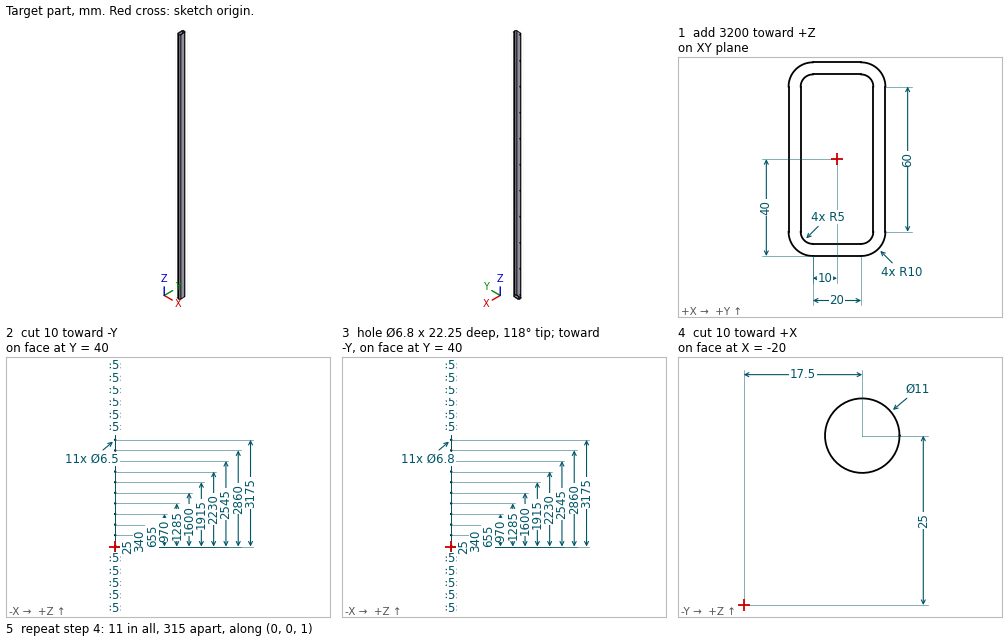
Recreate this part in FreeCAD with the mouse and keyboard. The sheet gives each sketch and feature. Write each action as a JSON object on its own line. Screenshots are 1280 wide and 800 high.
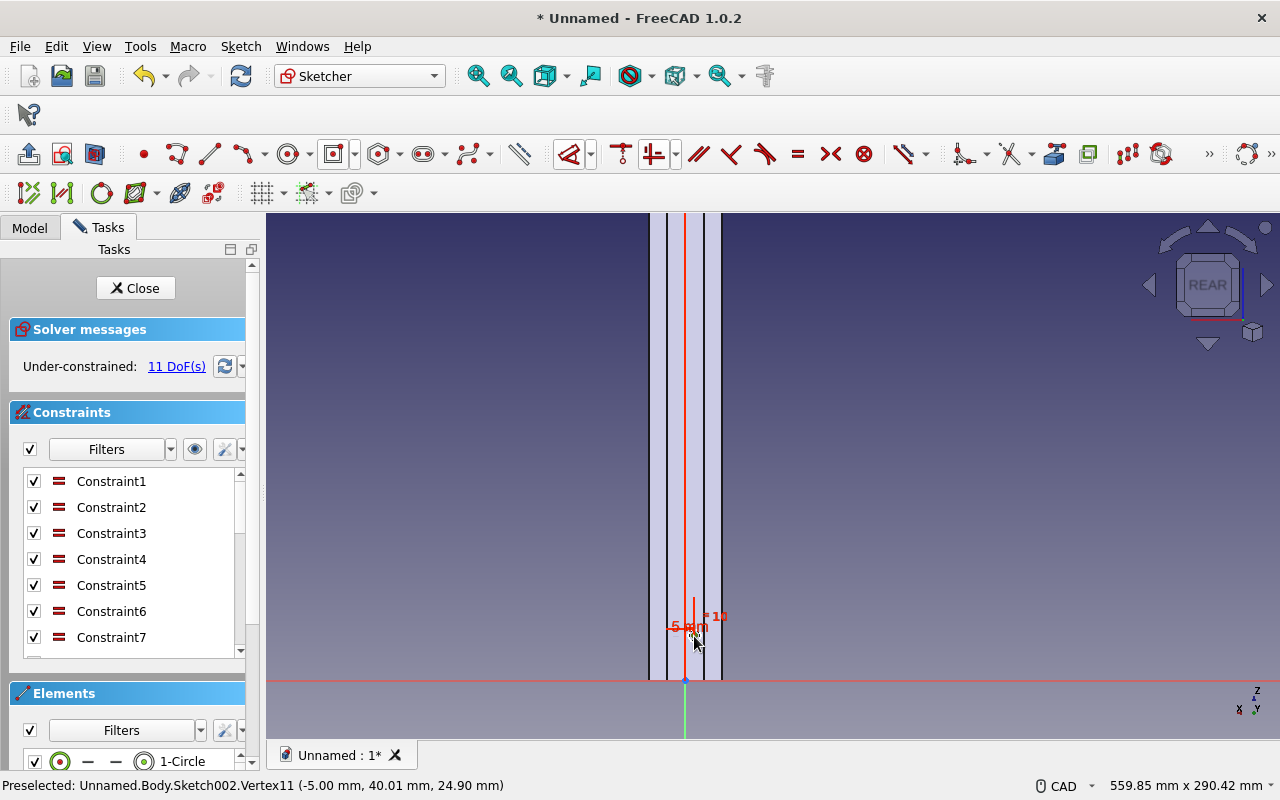
{"action": "key", "text": "i"}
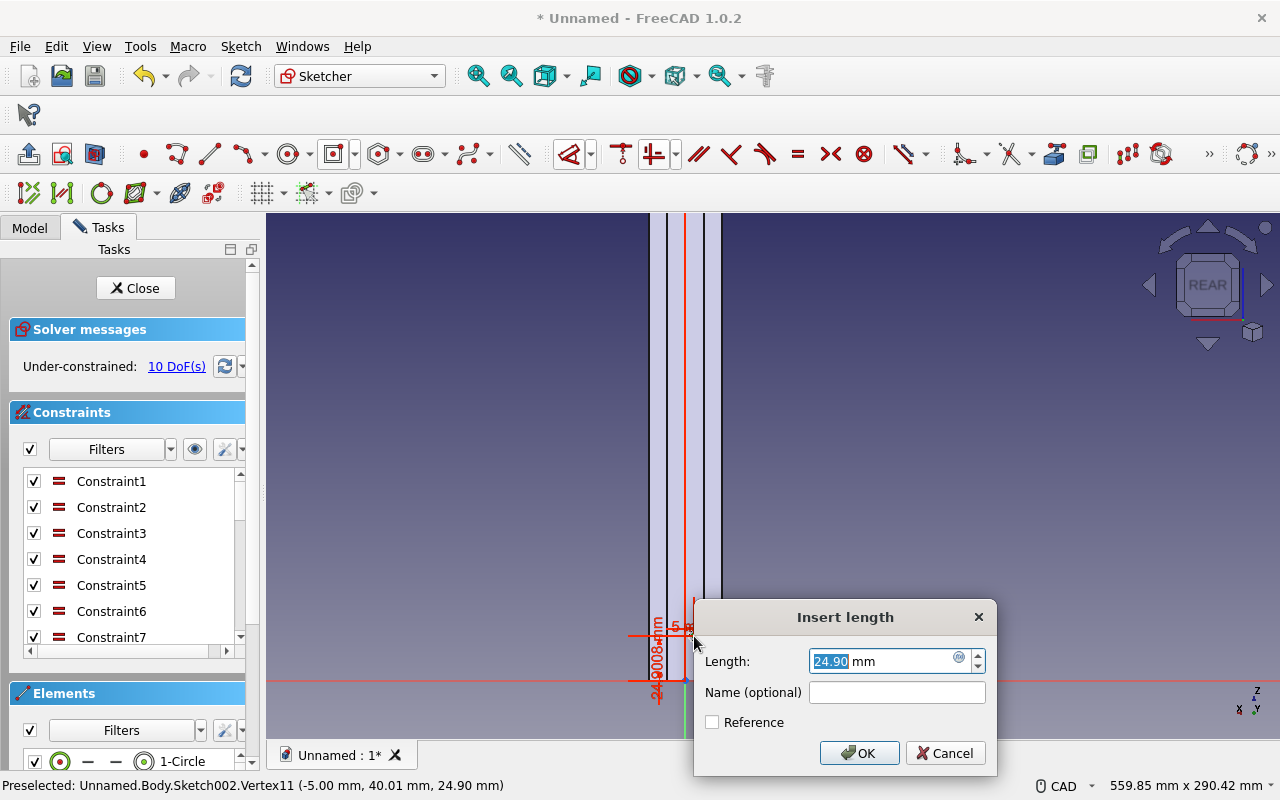
{"action": "type", "text": "25"}
{"action": "key", "text": "Return"}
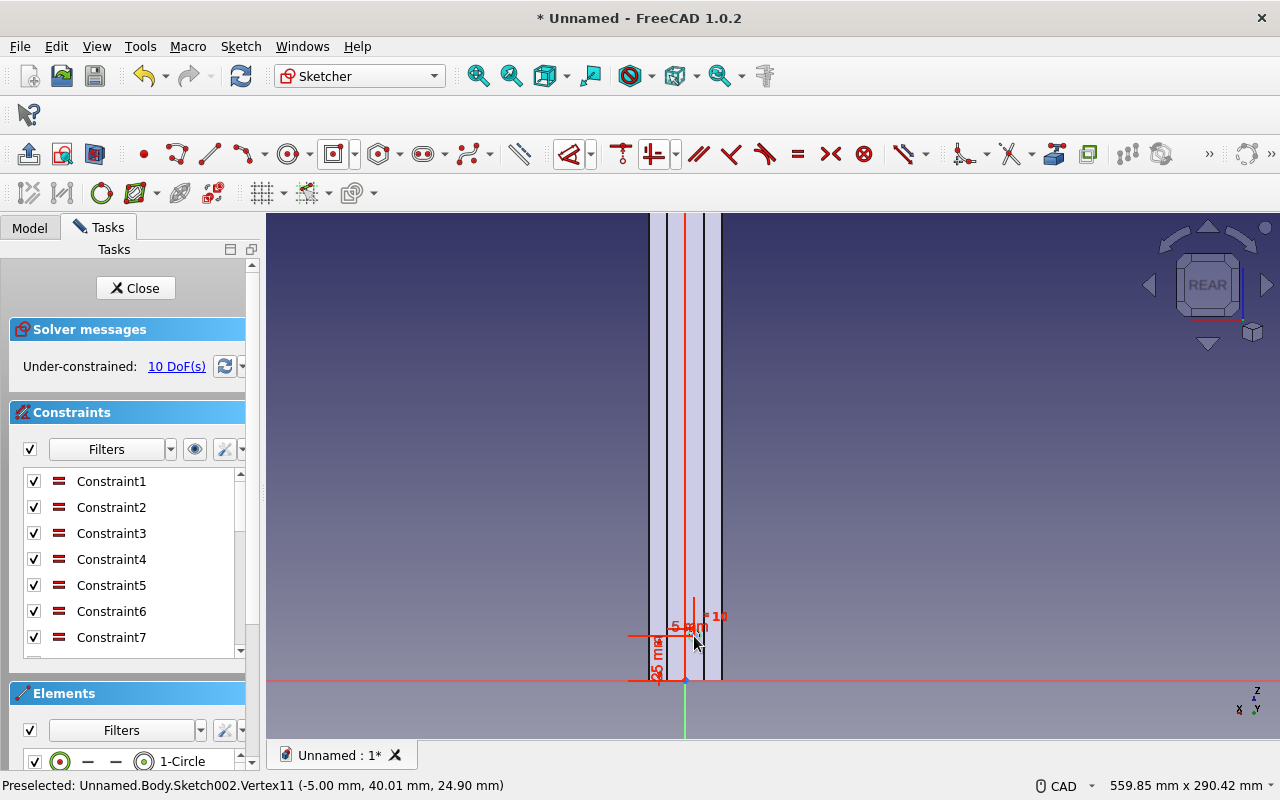
{"action": "scroll", "coordinate": [705, 649], "scroll_direction": "down", "scroll_amount": 14}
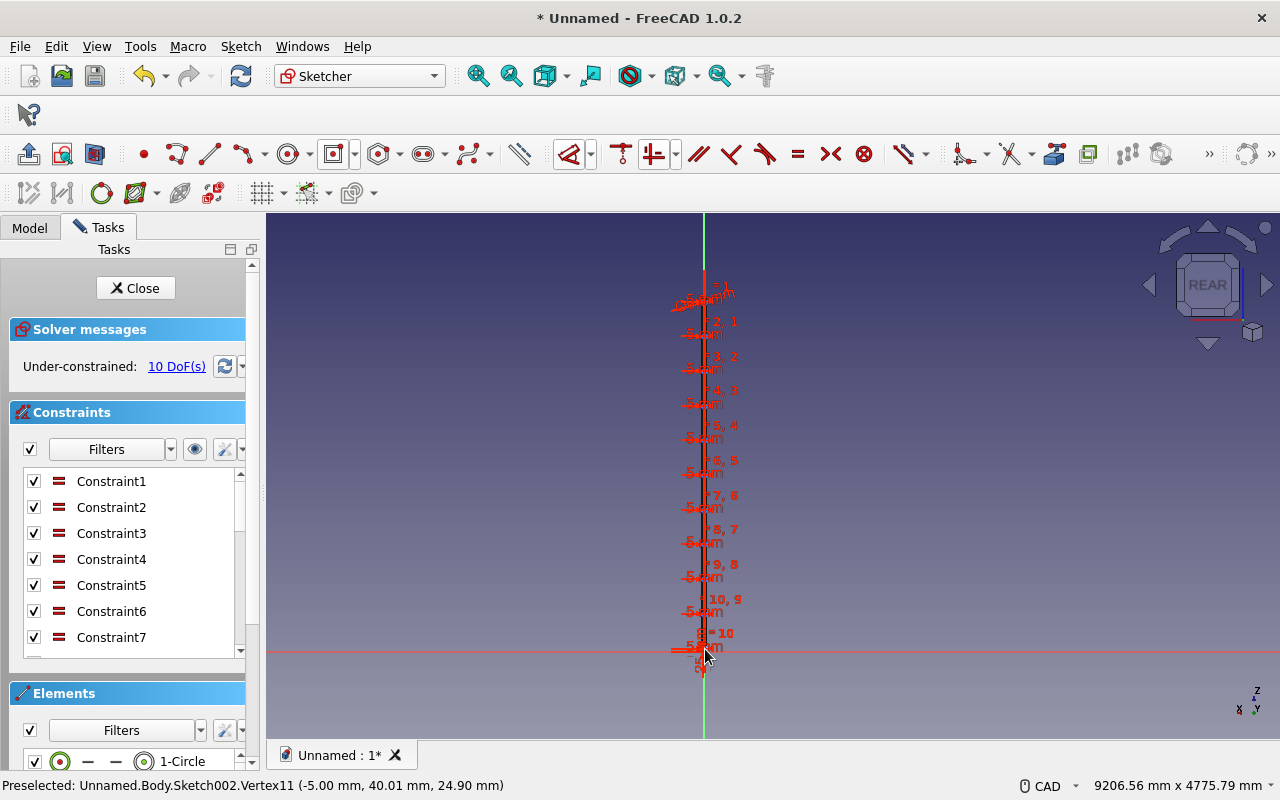
{"action": "left_click", "coordinate": [705, 545]}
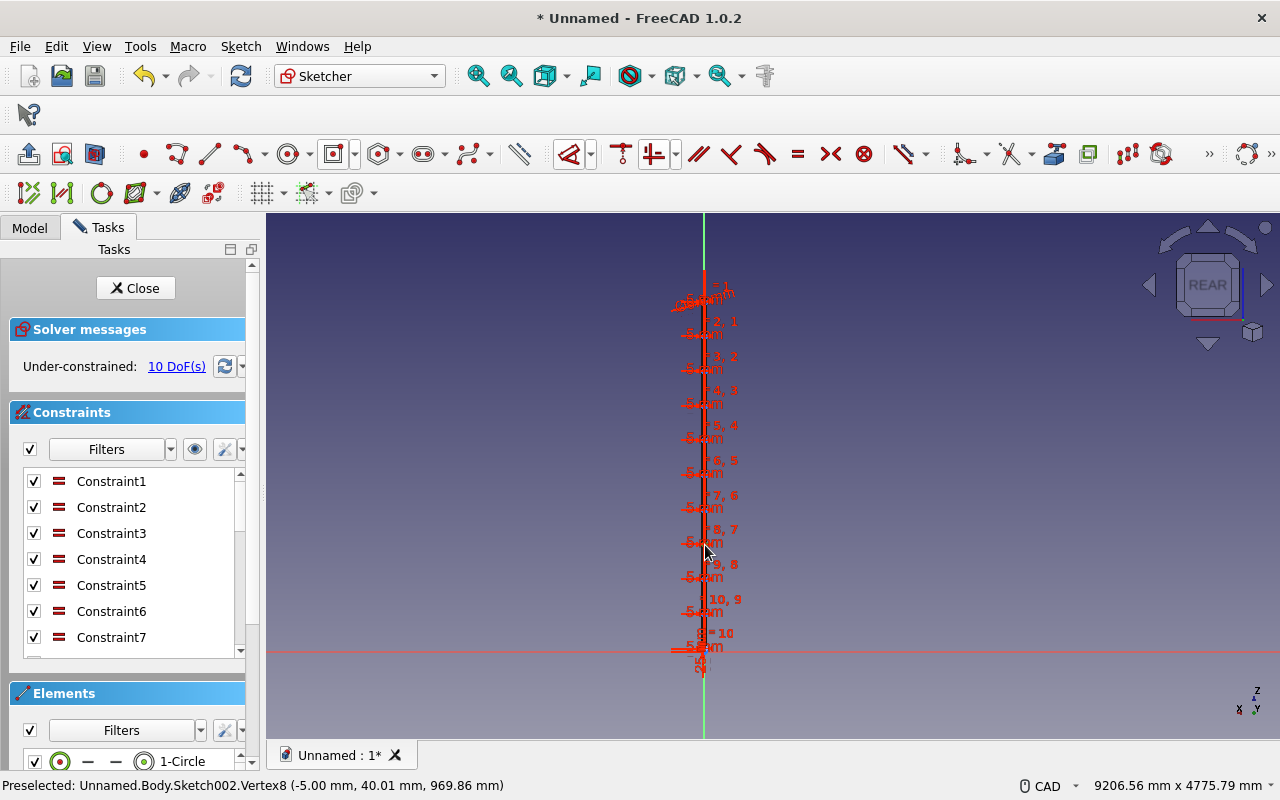
{"action": "key", "text": "i"}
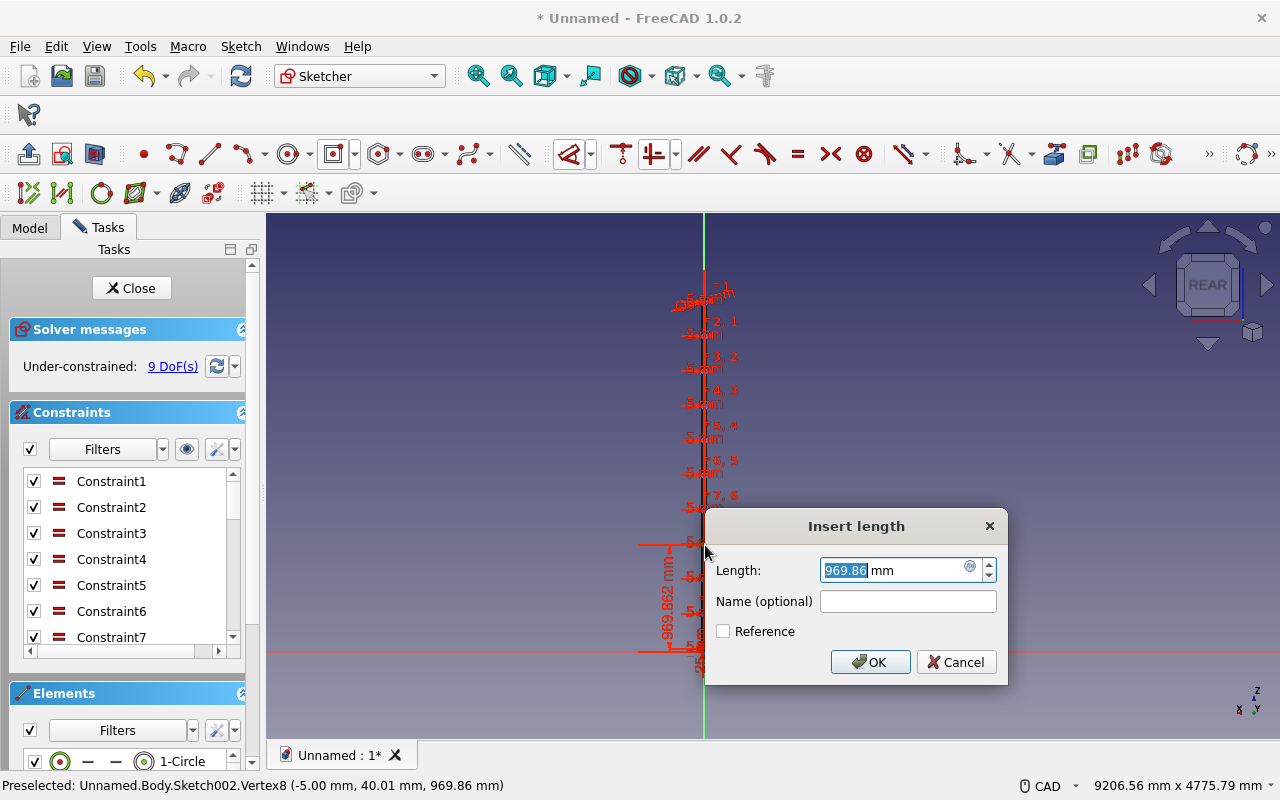
{"action": "type", "text": "970"}
{"action": "key", "text": "Return"}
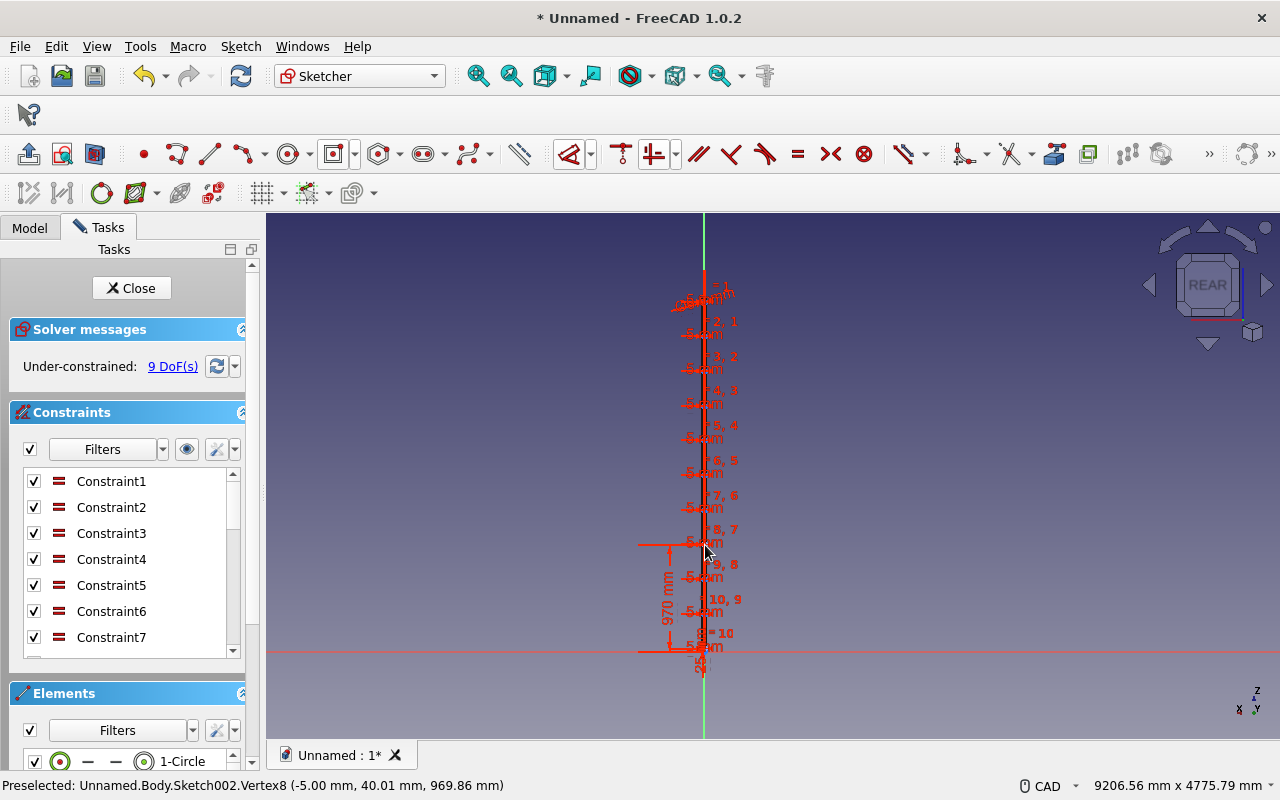
{"action": "left_click", "coordinate": [705, 580]}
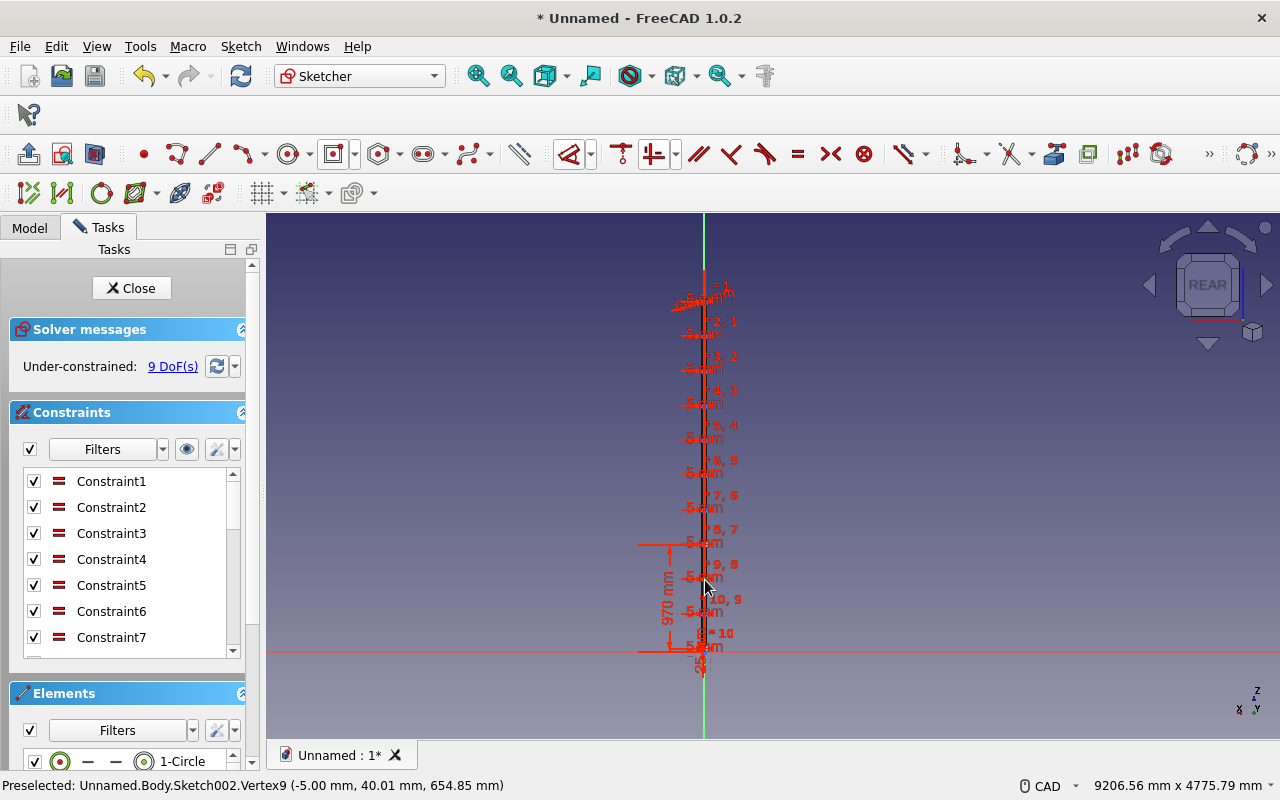
{"action": "left_click", "coordinate": [590, 154]}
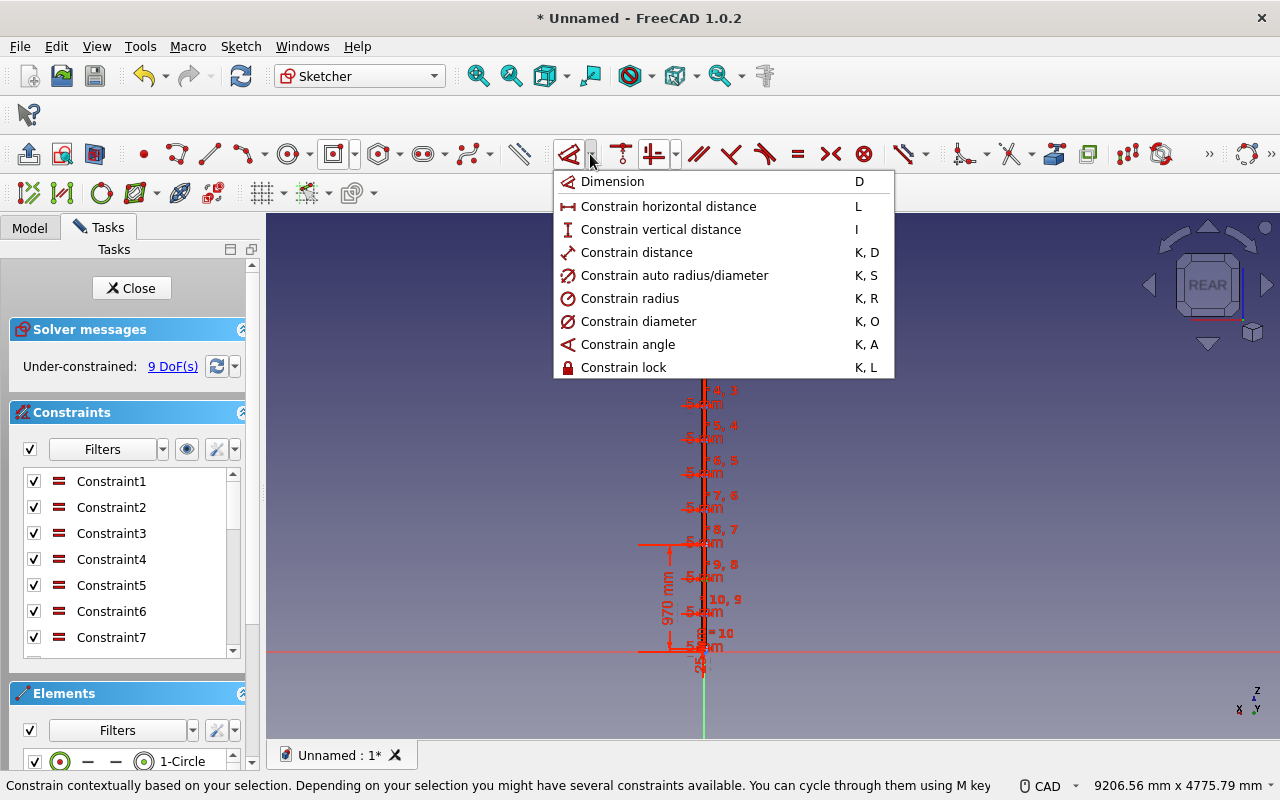
{"action": "left_click", "coordinate": [724, 230]}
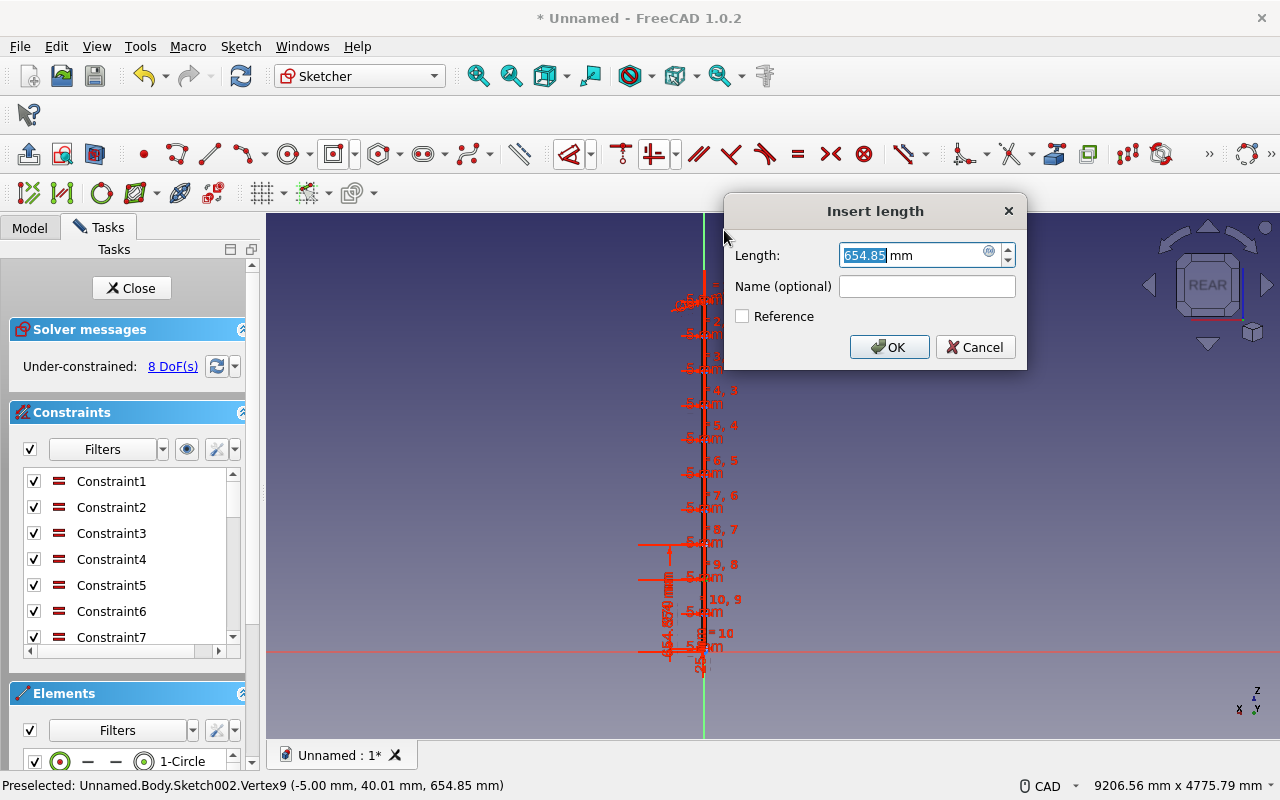
{"action": "type", "text": "655"}
{"action": "key", "text": "Return"}